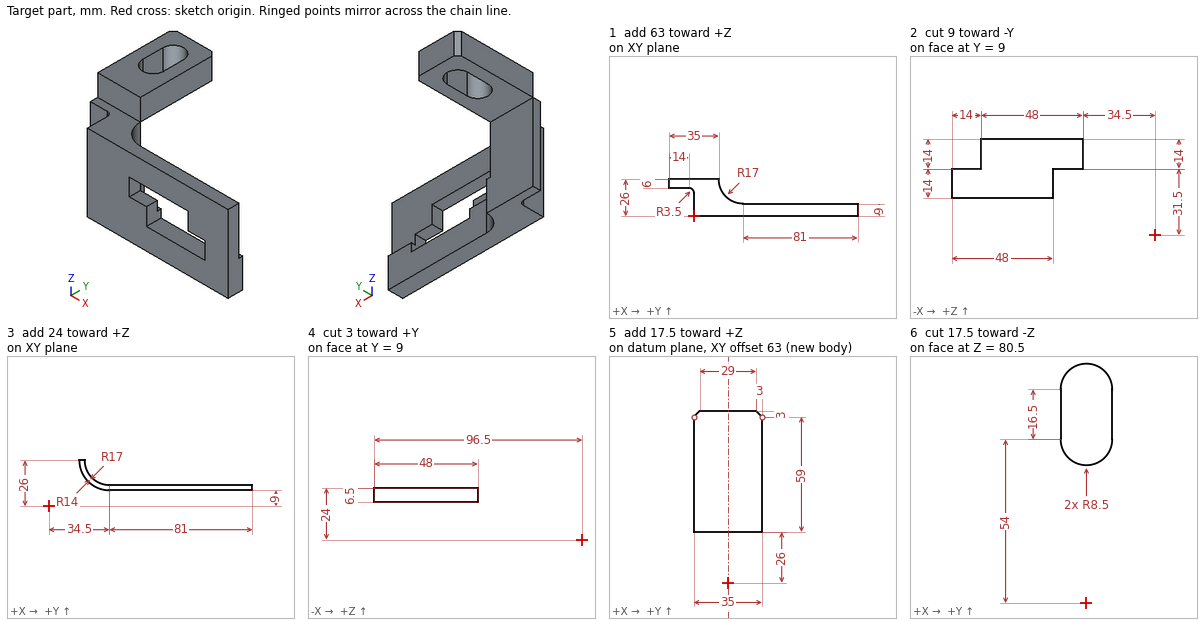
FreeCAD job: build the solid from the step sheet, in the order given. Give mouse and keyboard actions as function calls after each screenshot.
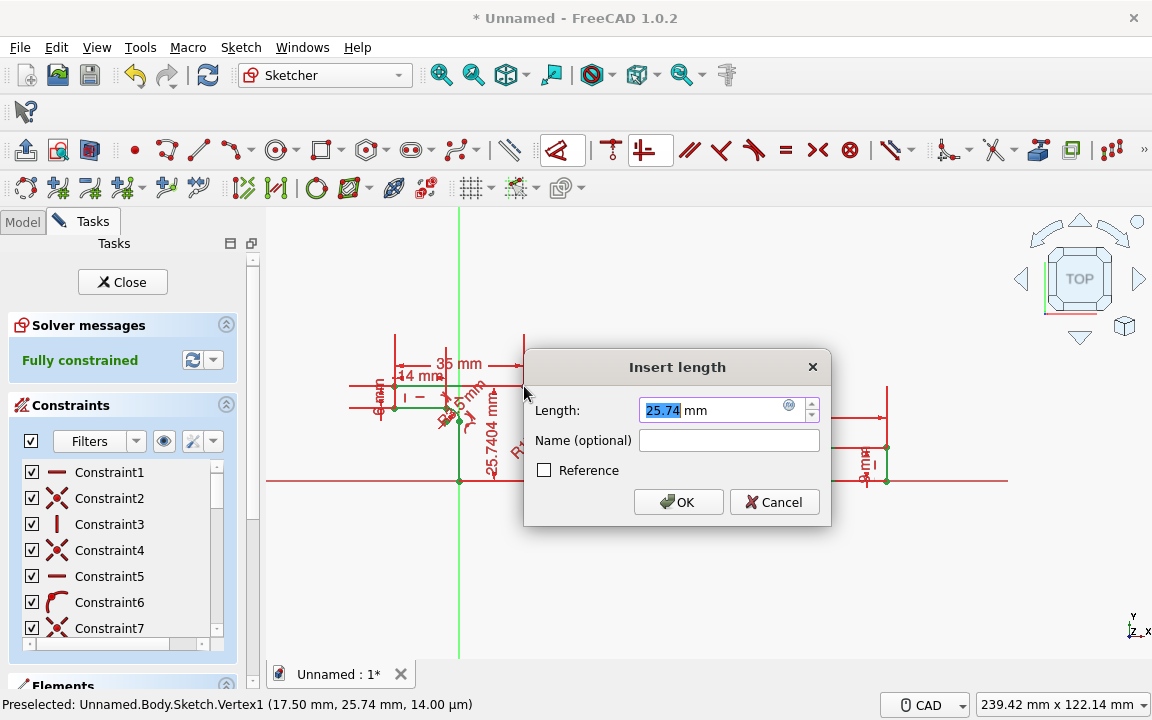
text(26)
key(Return)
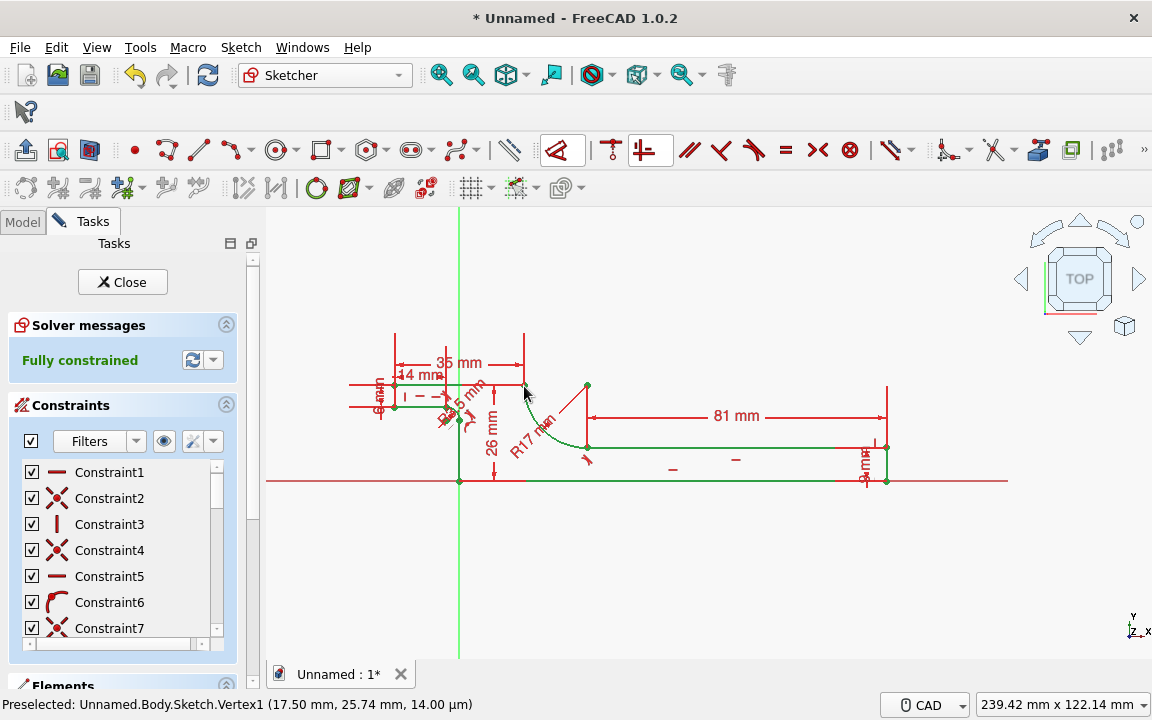
click(123, 282)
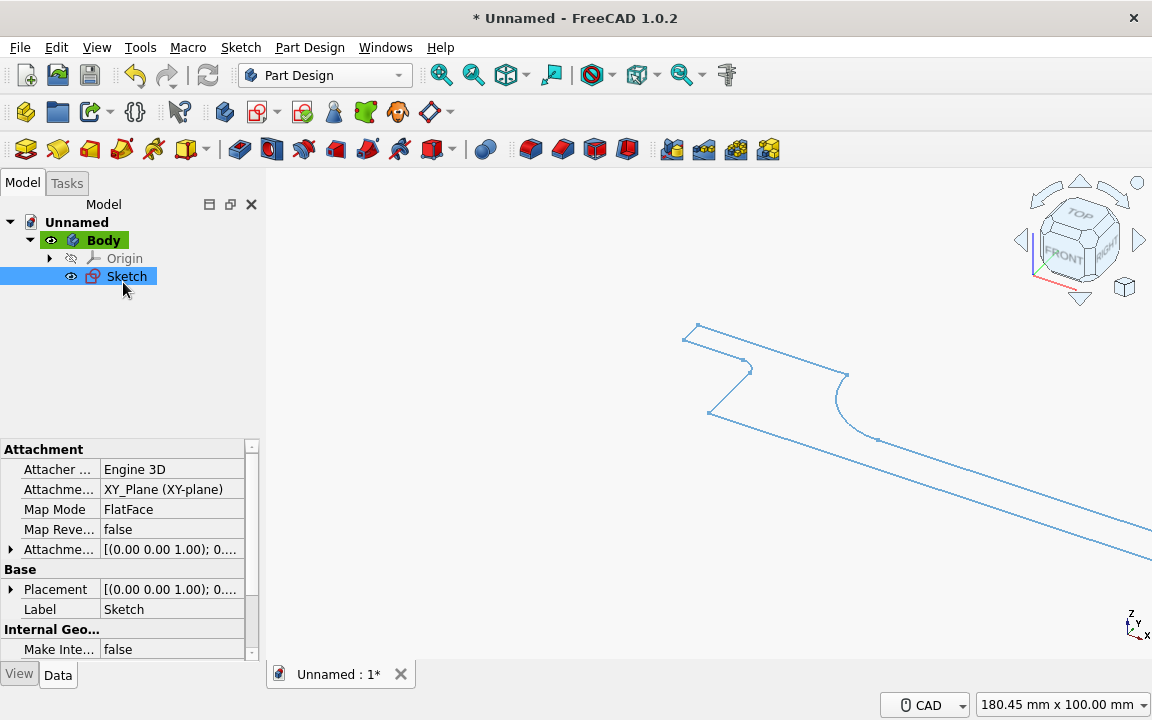
click(26, 150)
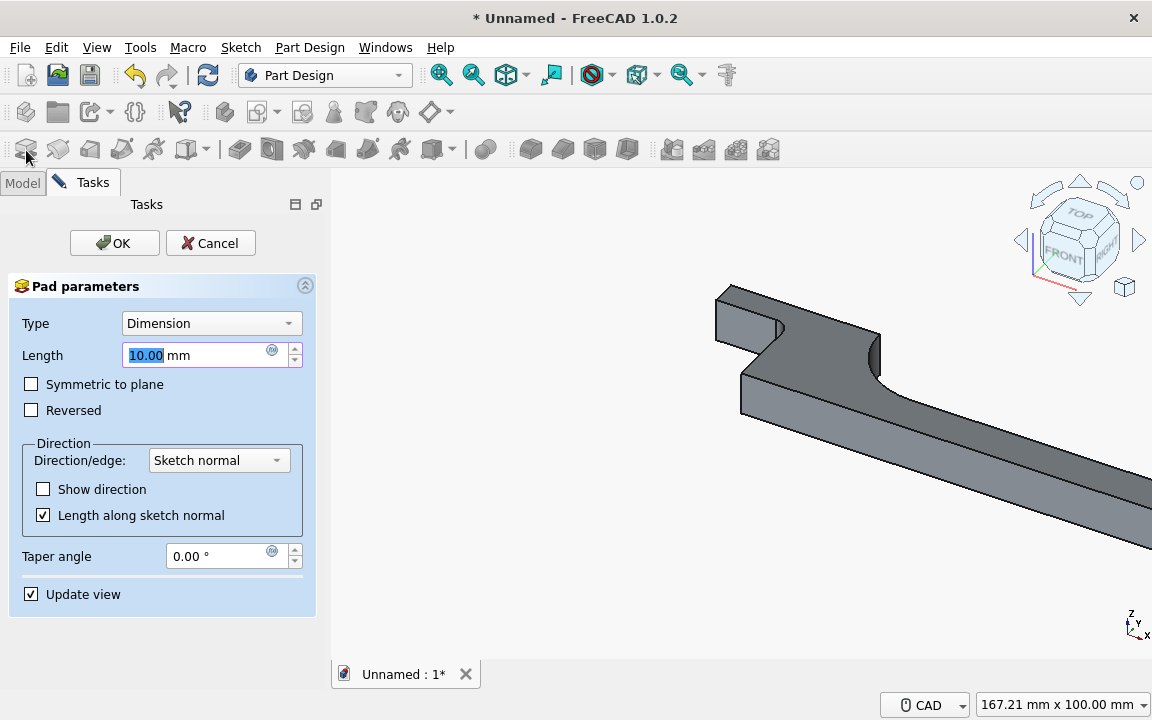
text(63)
key(Tab)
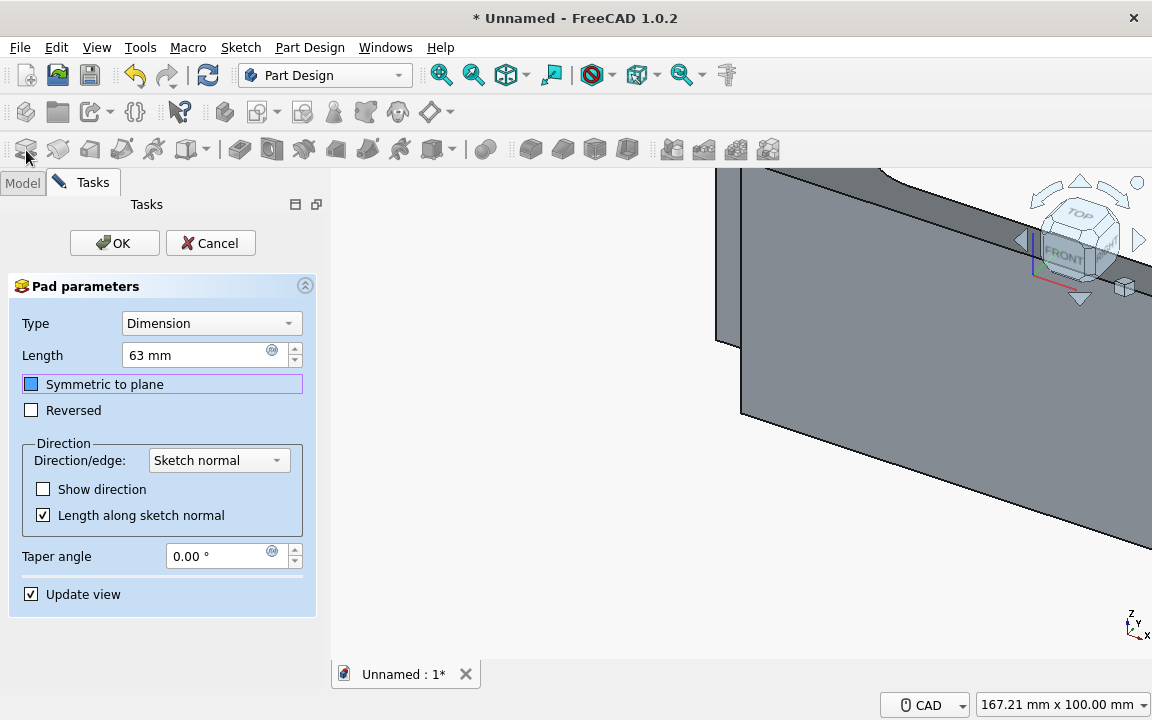
click(115, 243)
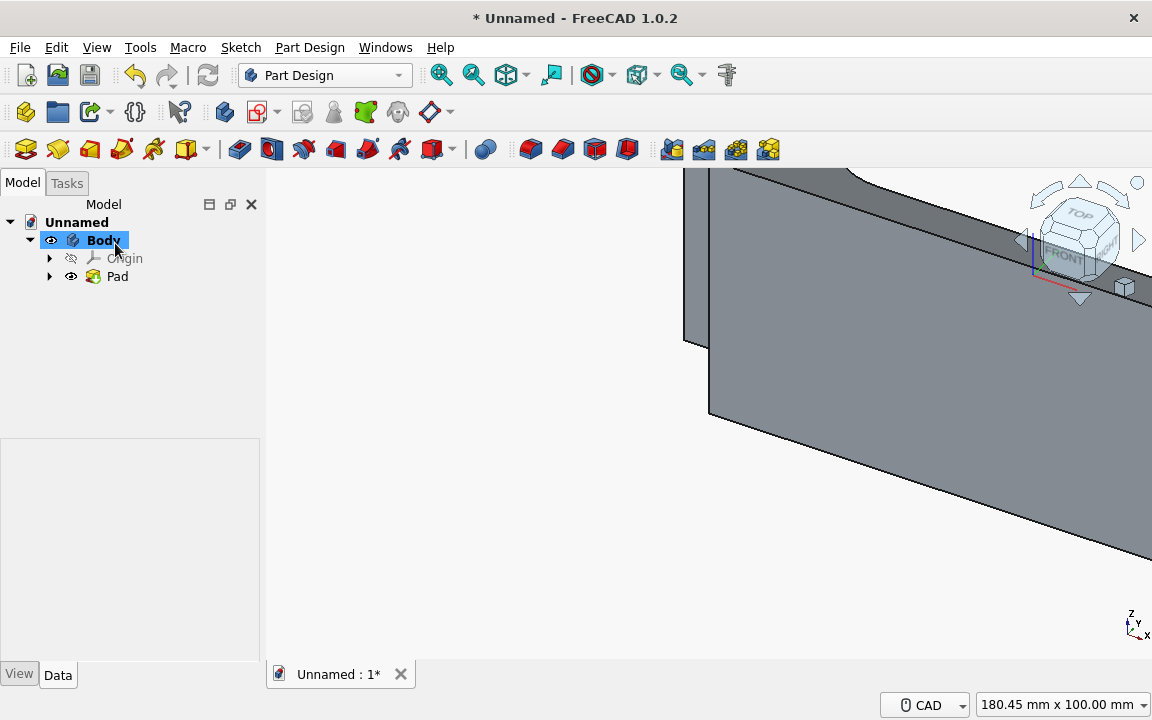
key(v)
key(f)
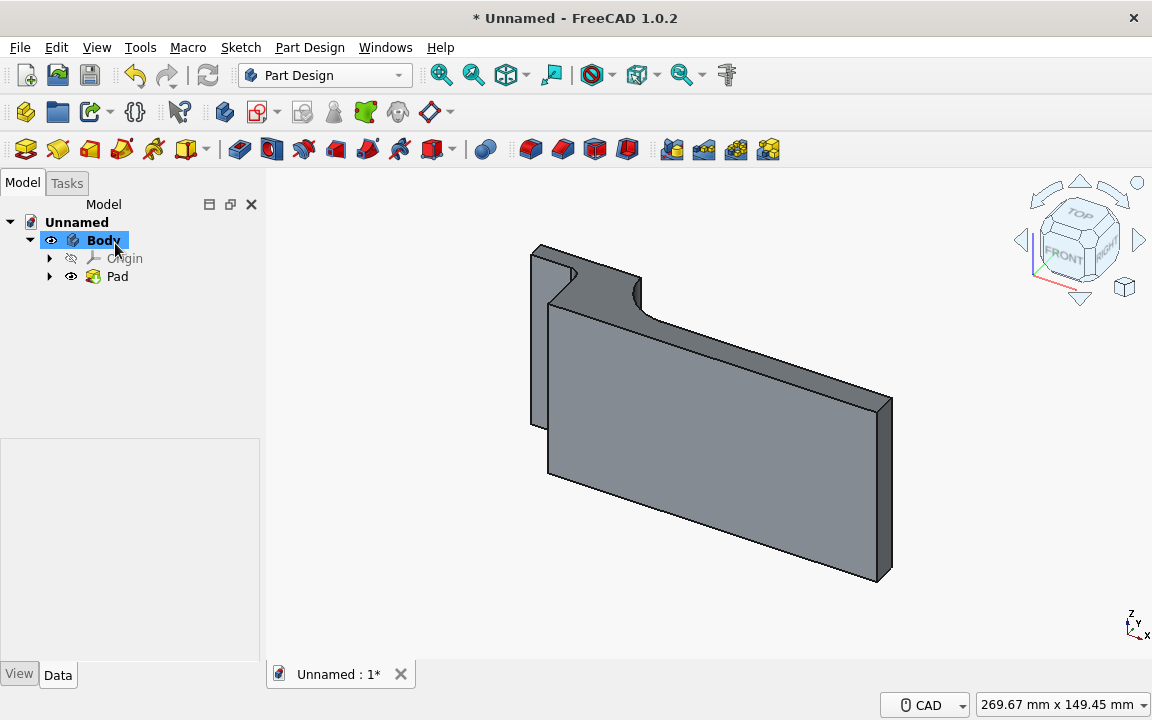
key(4)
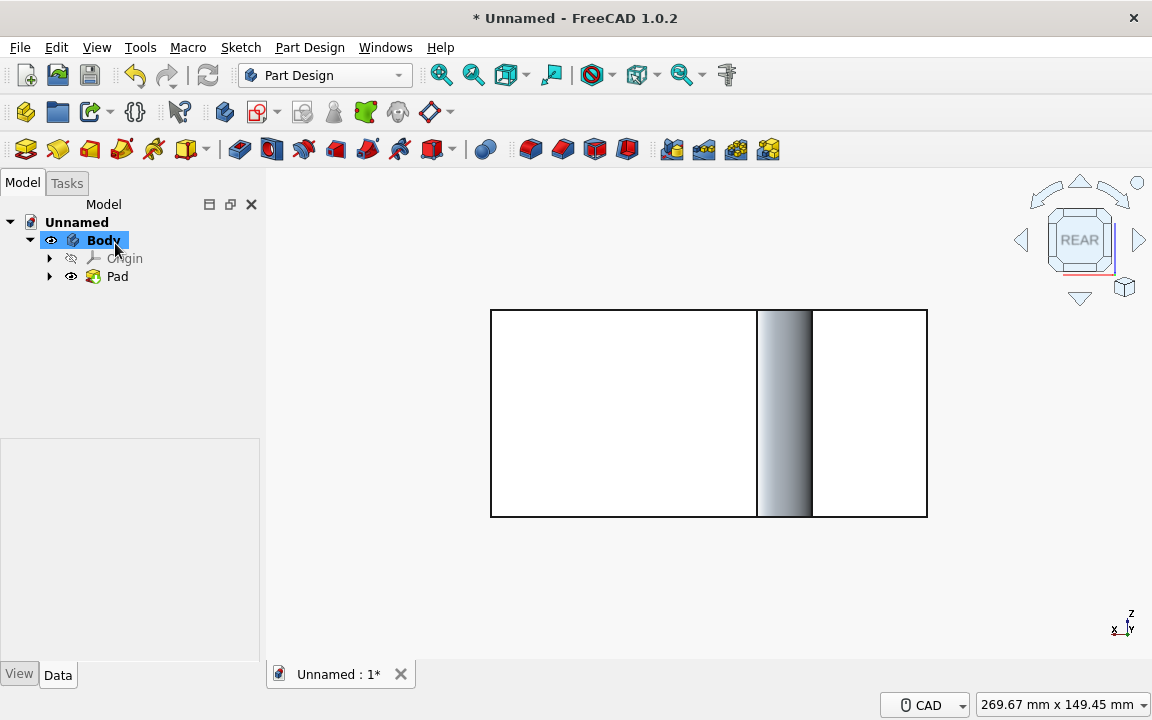
click(624, 413)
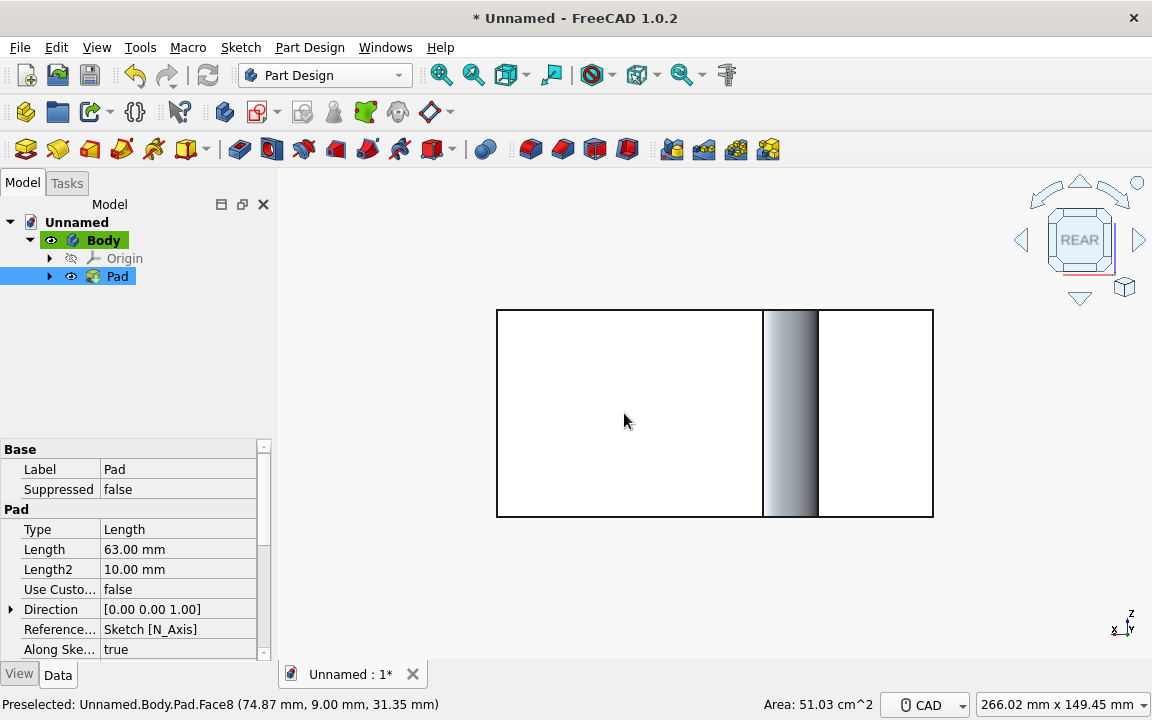
click(258, 112)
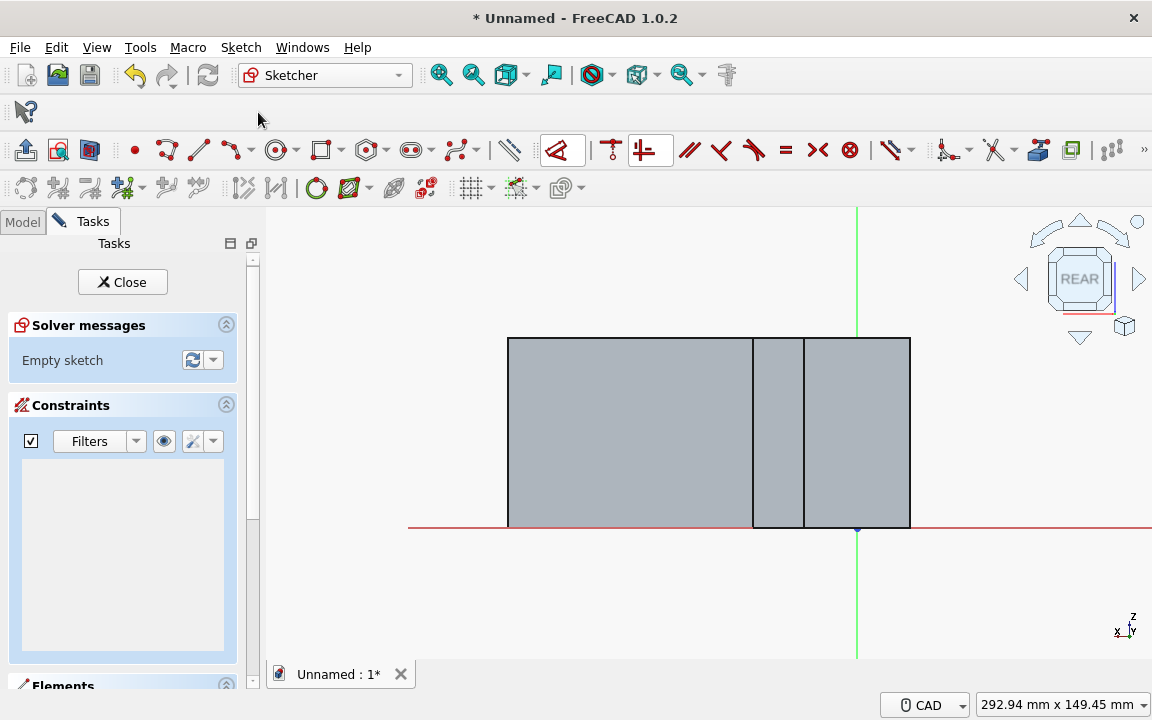
click(90, 150)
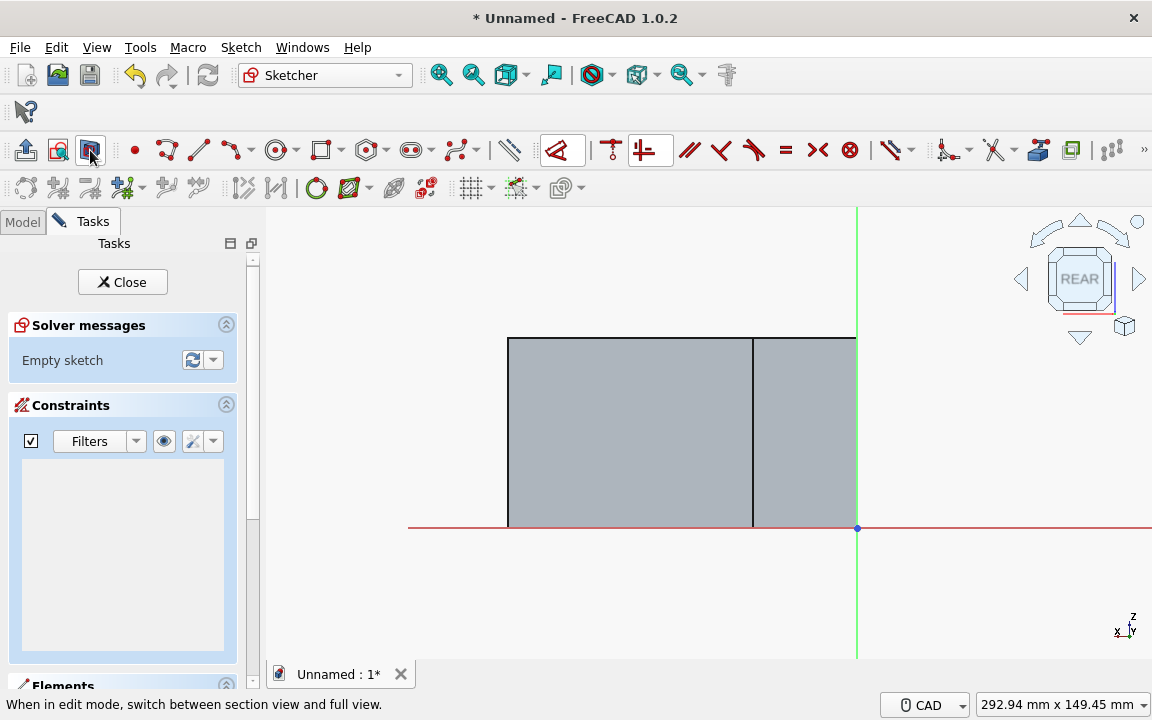
scroll(797, 492, up, 3)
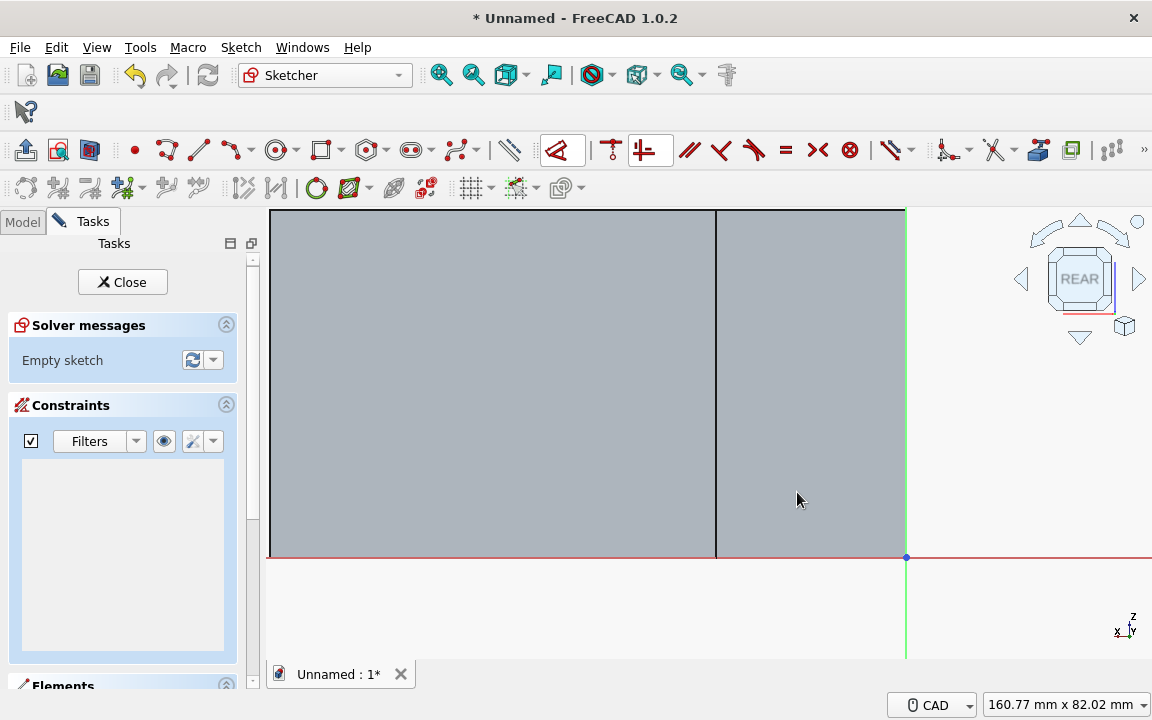
key(g)
key(m)